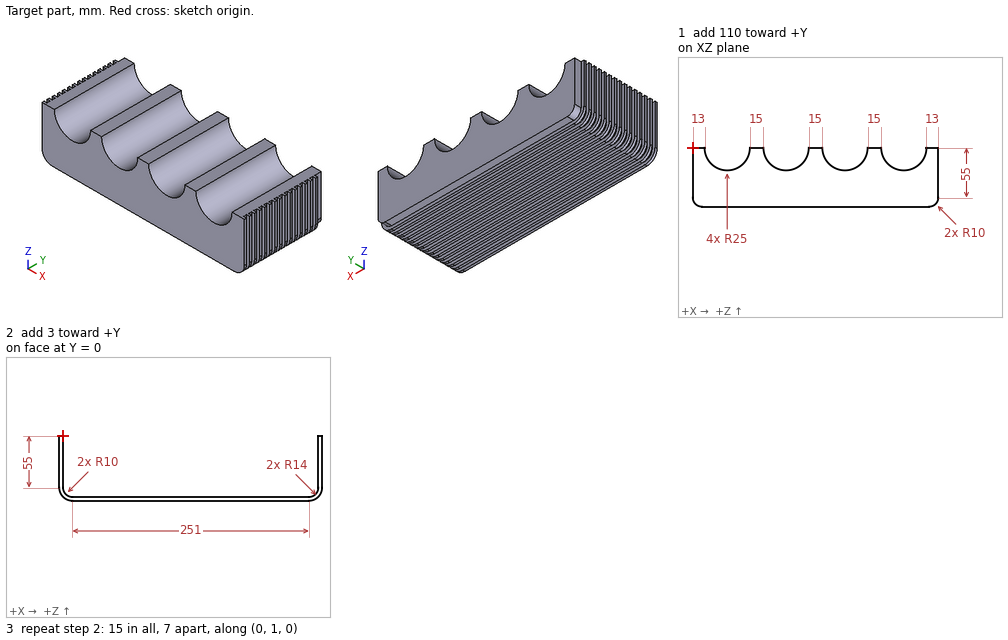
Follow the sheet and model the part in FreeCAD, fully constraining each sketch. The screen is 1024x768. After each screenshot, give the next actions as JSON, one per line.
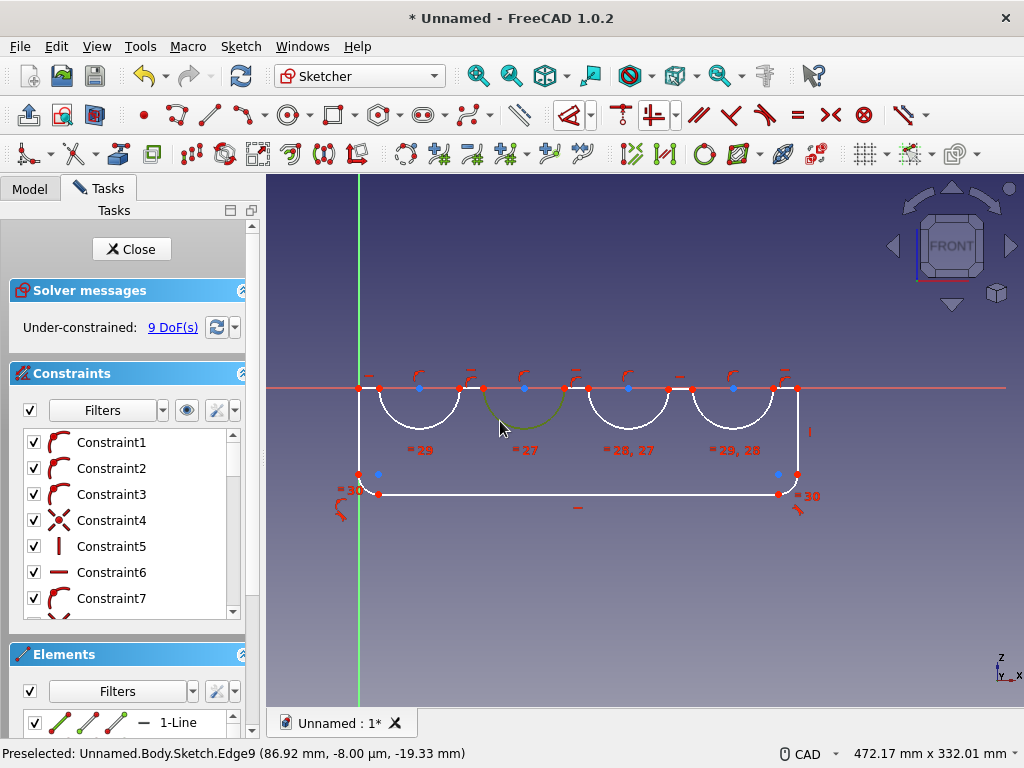
{"action": "left_click", "coordinate": [590, 116]}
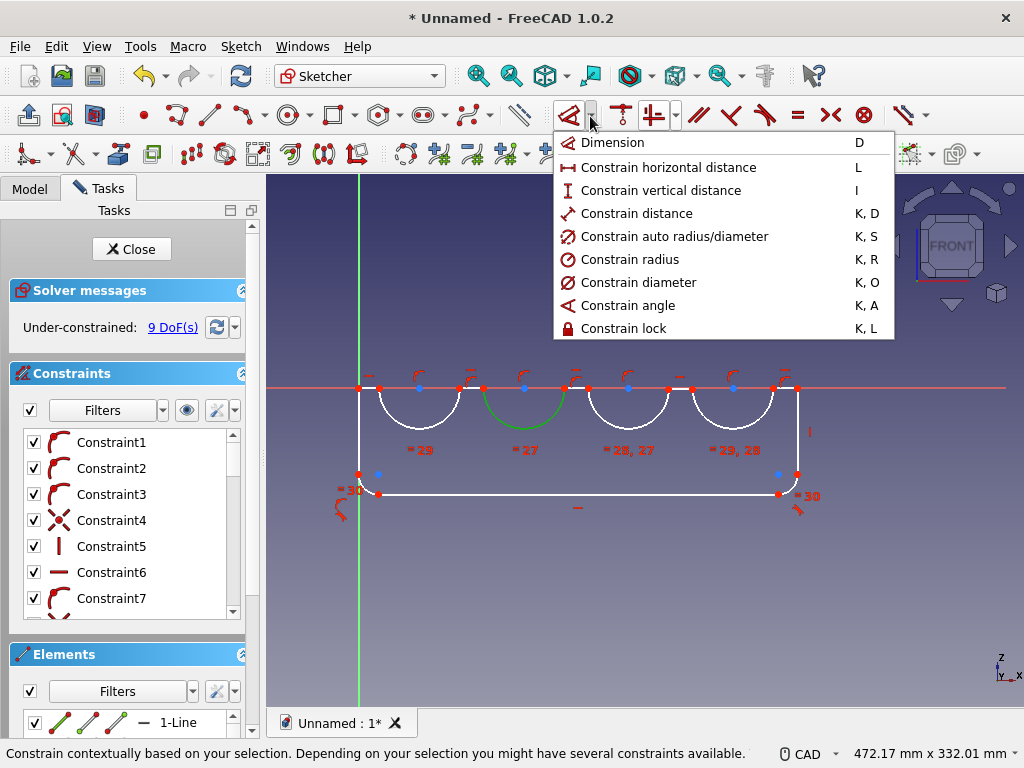
{"action": "left_click", "coordinate": [724, 260]}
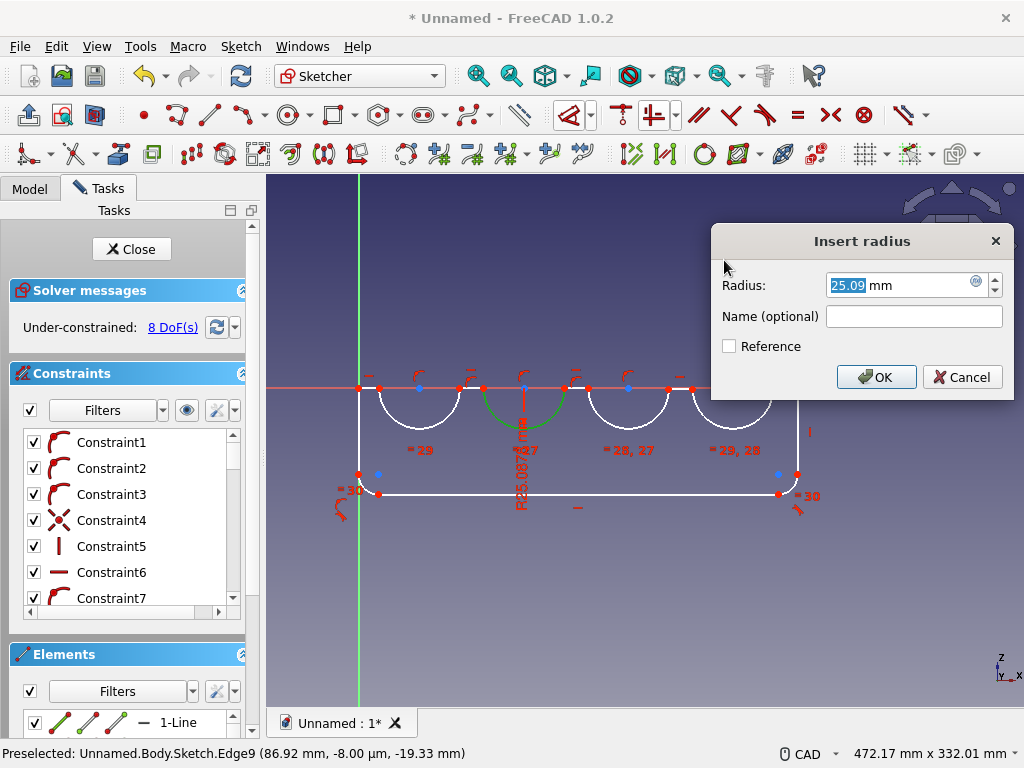
{"action": "type", "text": "25"}
{"action": "key", "text": "Return"}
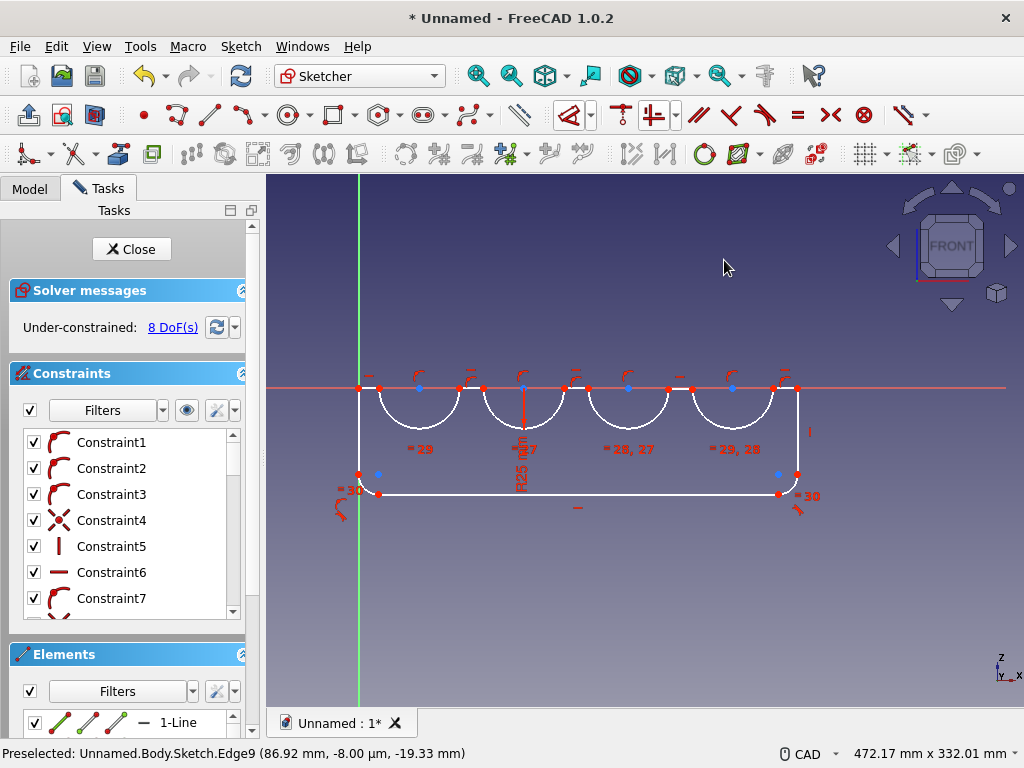
{"action": "scroll", "coordinate": [787, 492], "scroll_direction": "up", "scroll_amount": 5}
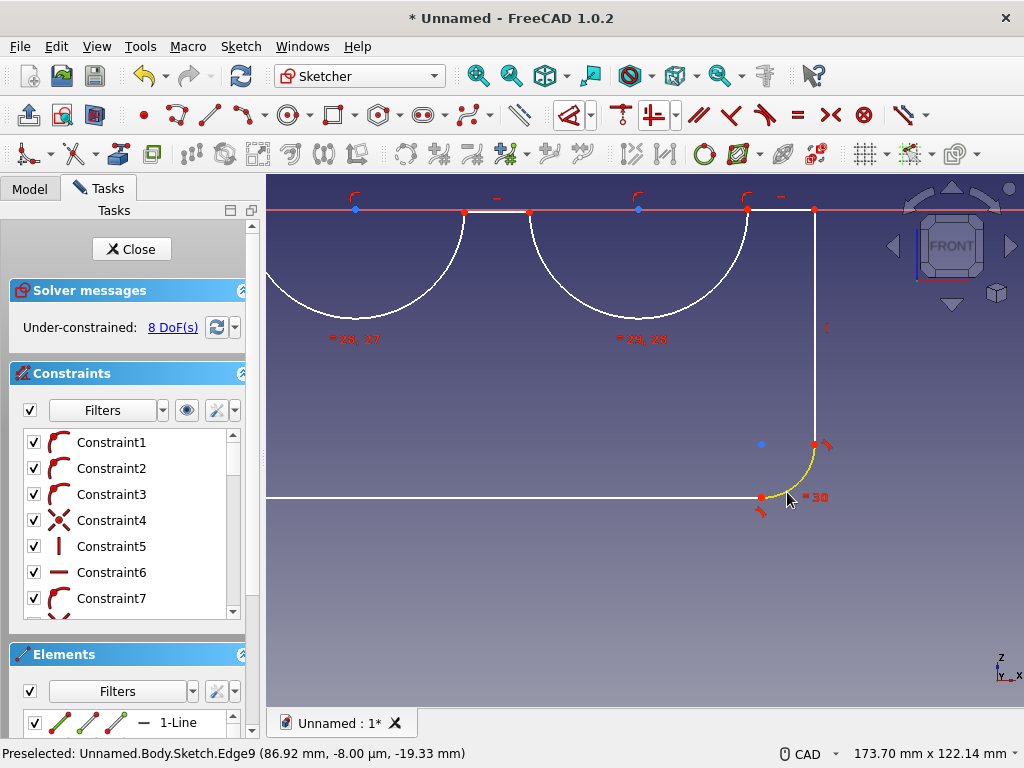
{"action": "left_click", "coordinate": [786, 492]}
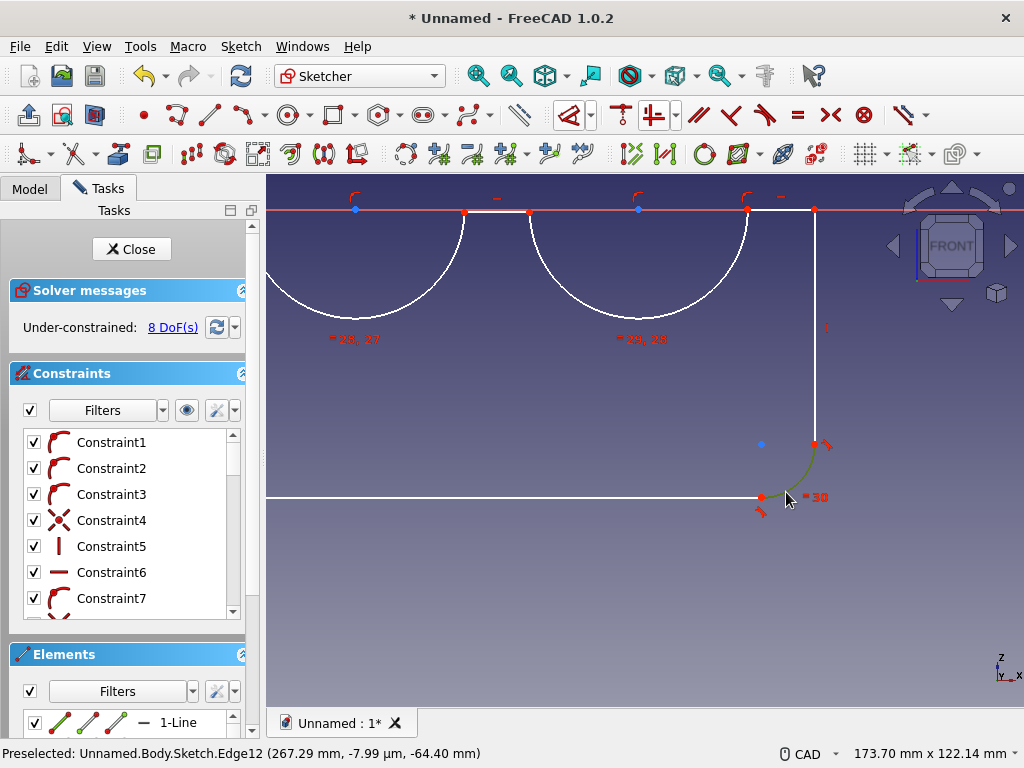
{"action": "key", "text": "k r"}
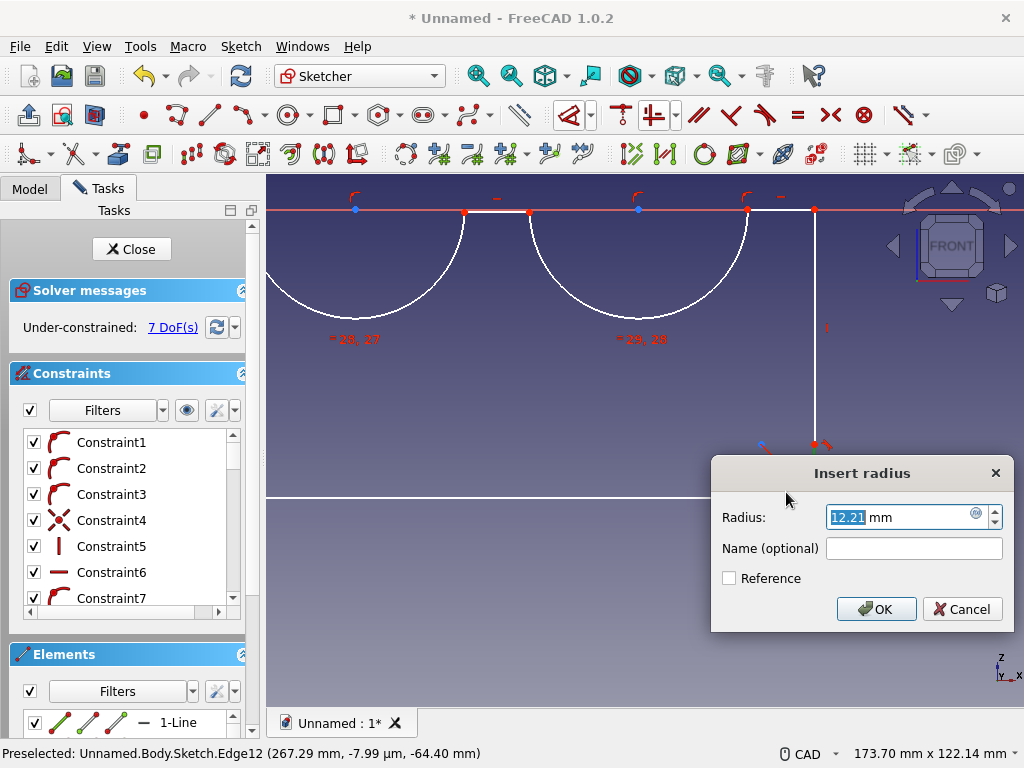
{"action": "type", "text": "10"}
{"action": "key", "text": "Return"}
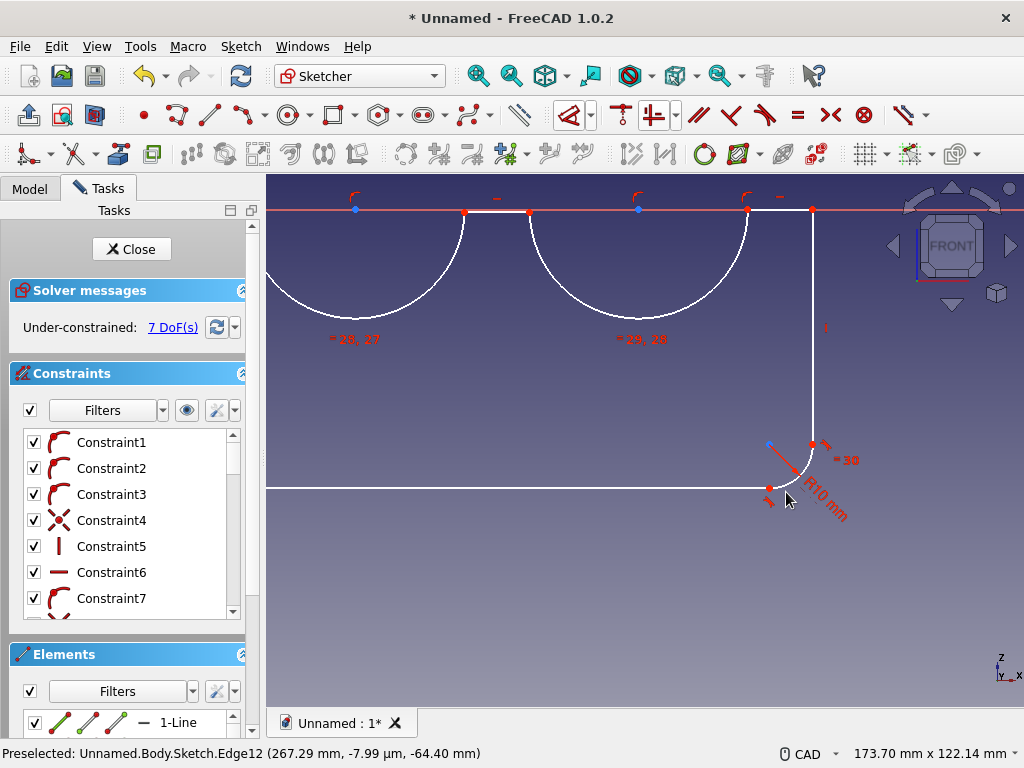
{"action": "left_click", "coordinate": [464, 212]}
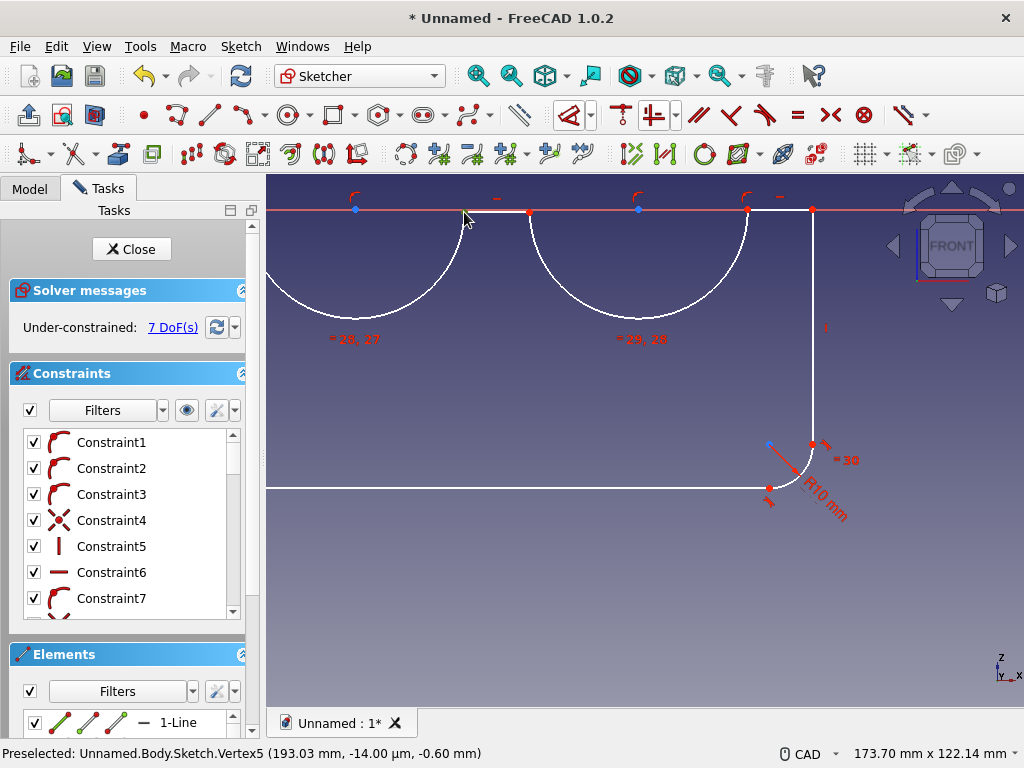
{"action": "left_click", "coordinate": [334, 210]}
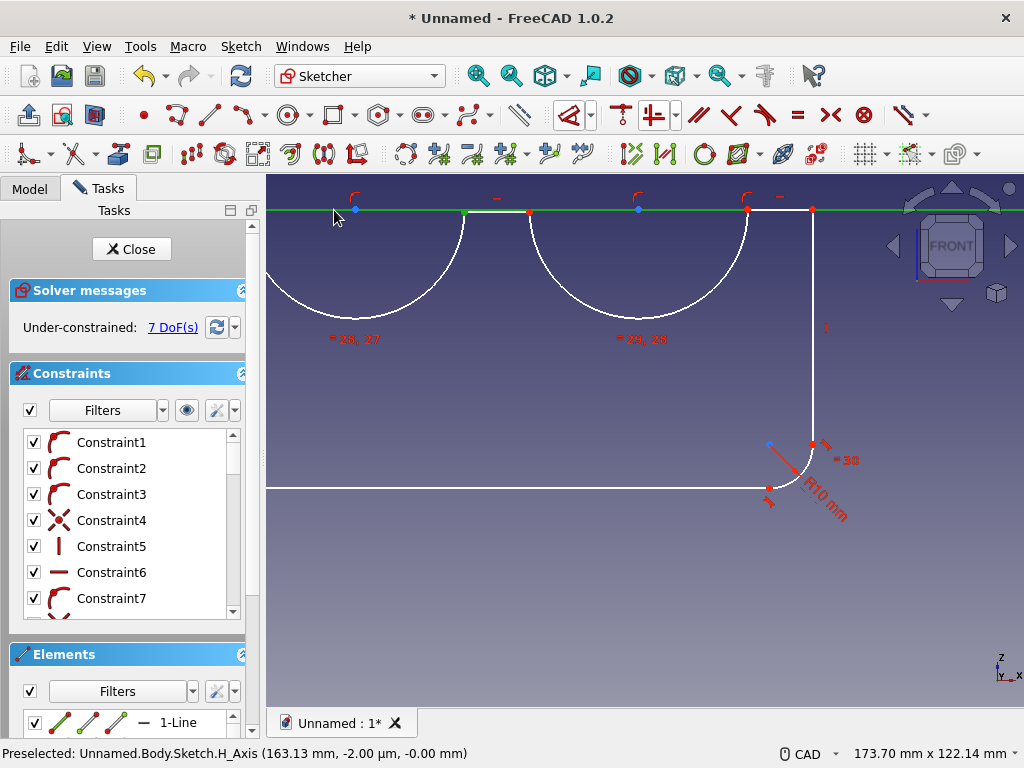
{"action": "key", "text": "c"}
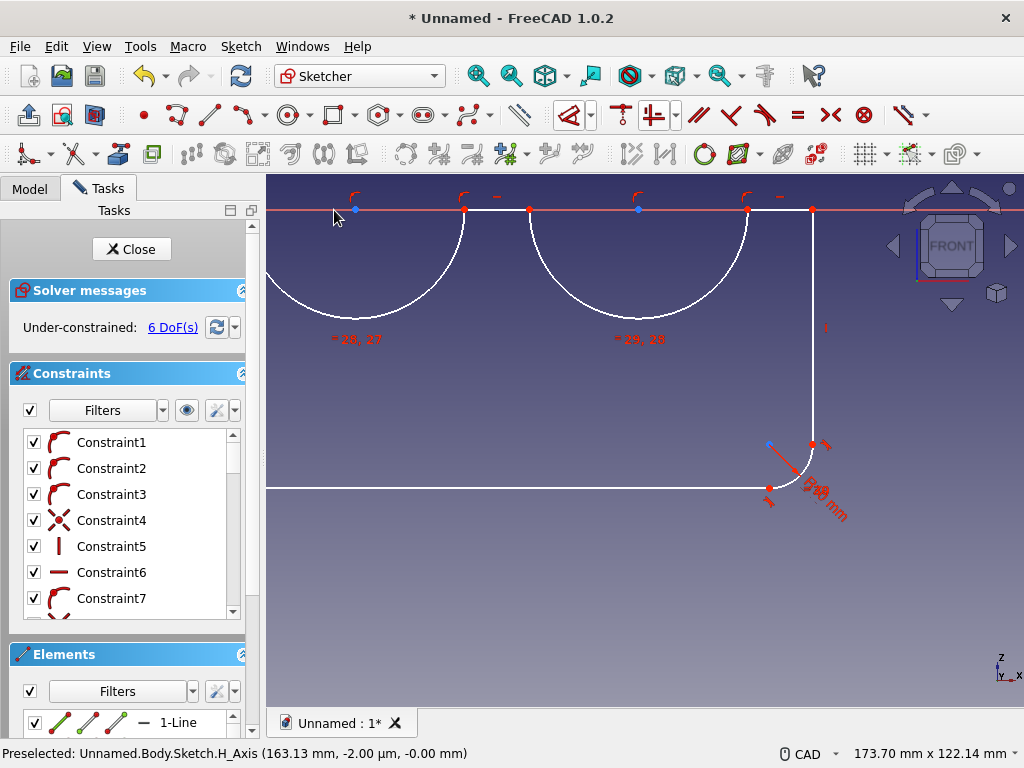
{"action": "scroll", "coordinate": [788, 492], "scroll_direction": "down", "scroll_amount": 5}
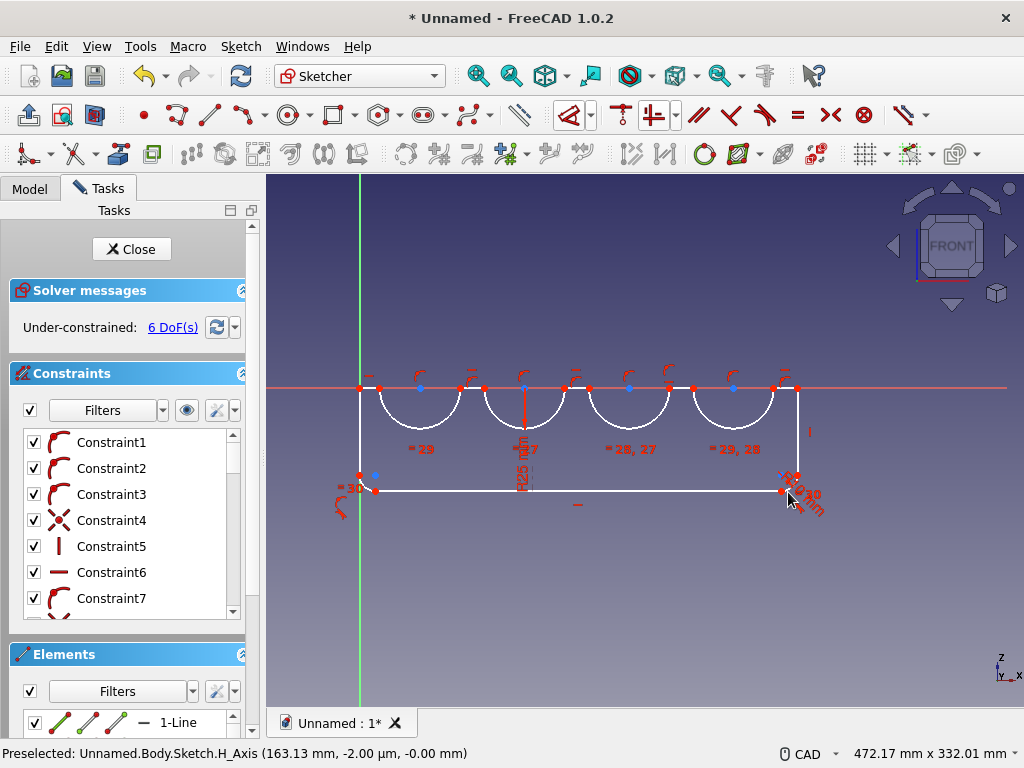
{"action": "scroll", "coordinate": [467, 388], "scroll_direction": "up", "scroll_amount": 4}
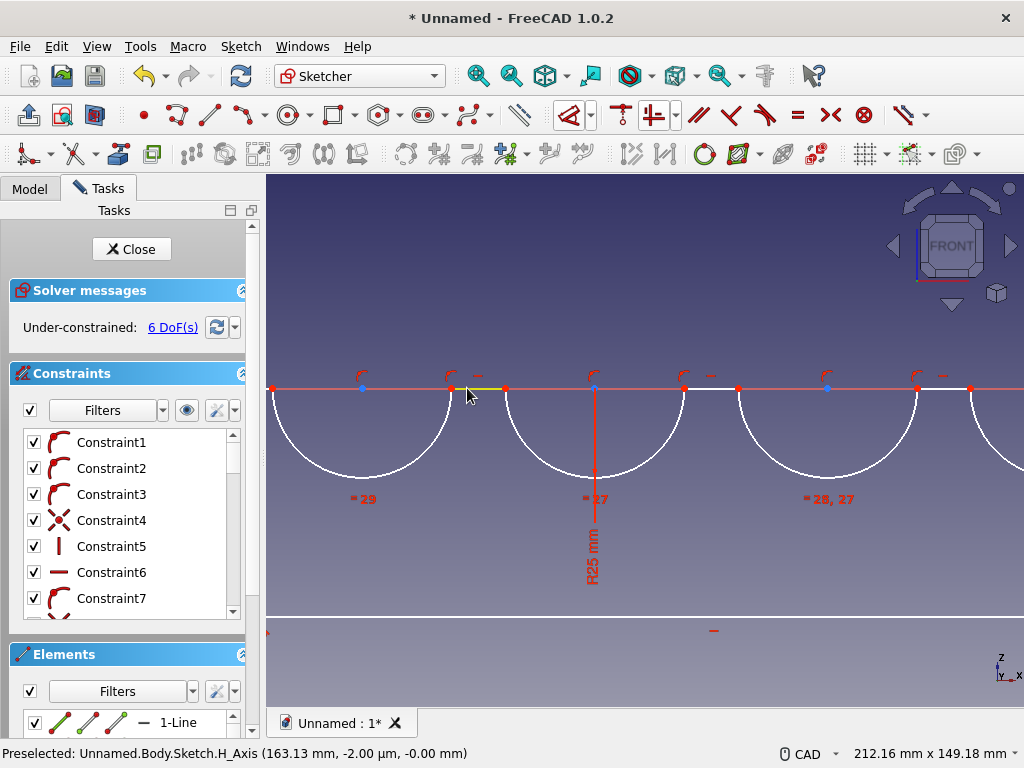
{"action": "left_click", "coordinate": [468, 389]}